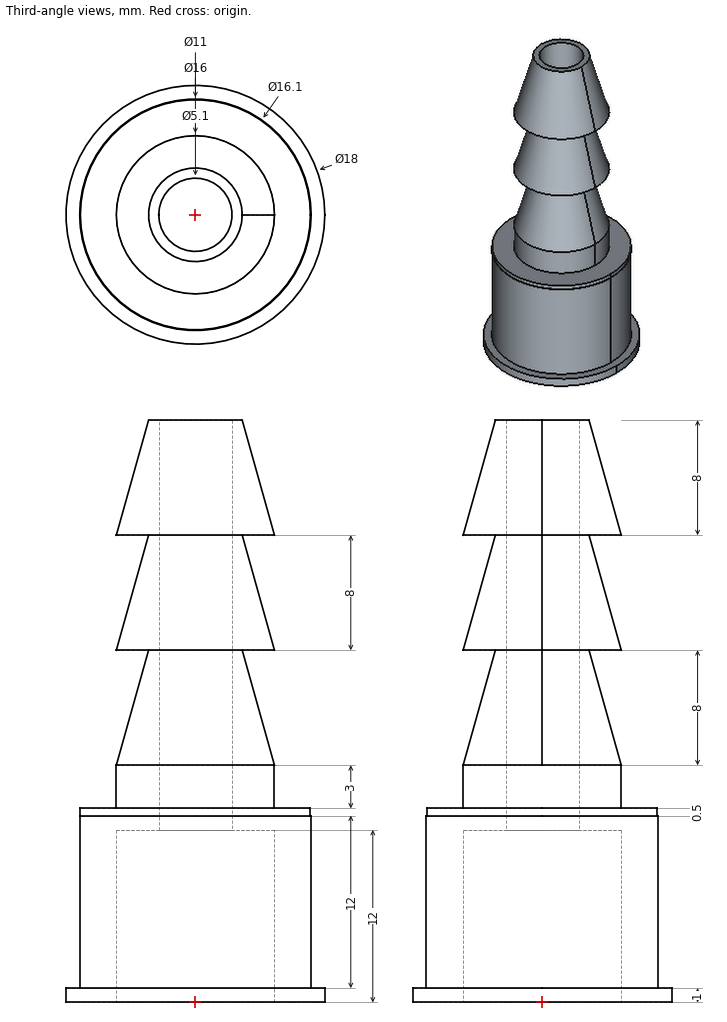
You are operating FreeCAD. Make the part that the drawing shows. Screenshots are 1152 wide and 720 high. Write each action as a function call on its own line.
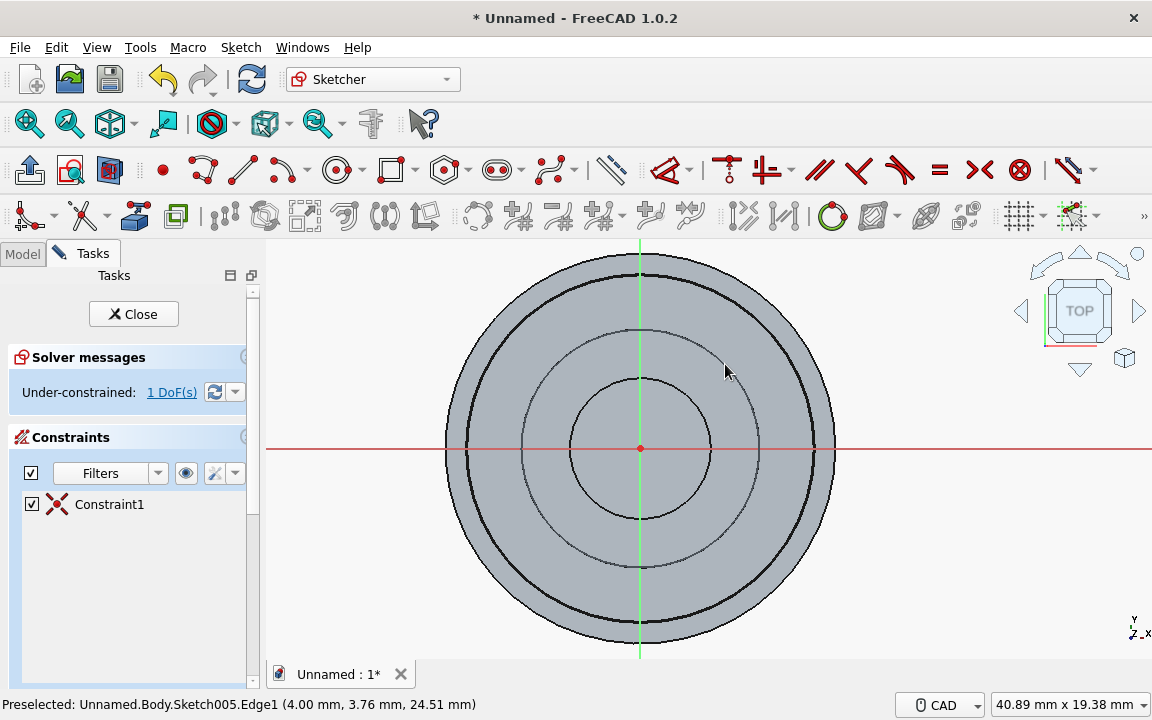
click(666, 170)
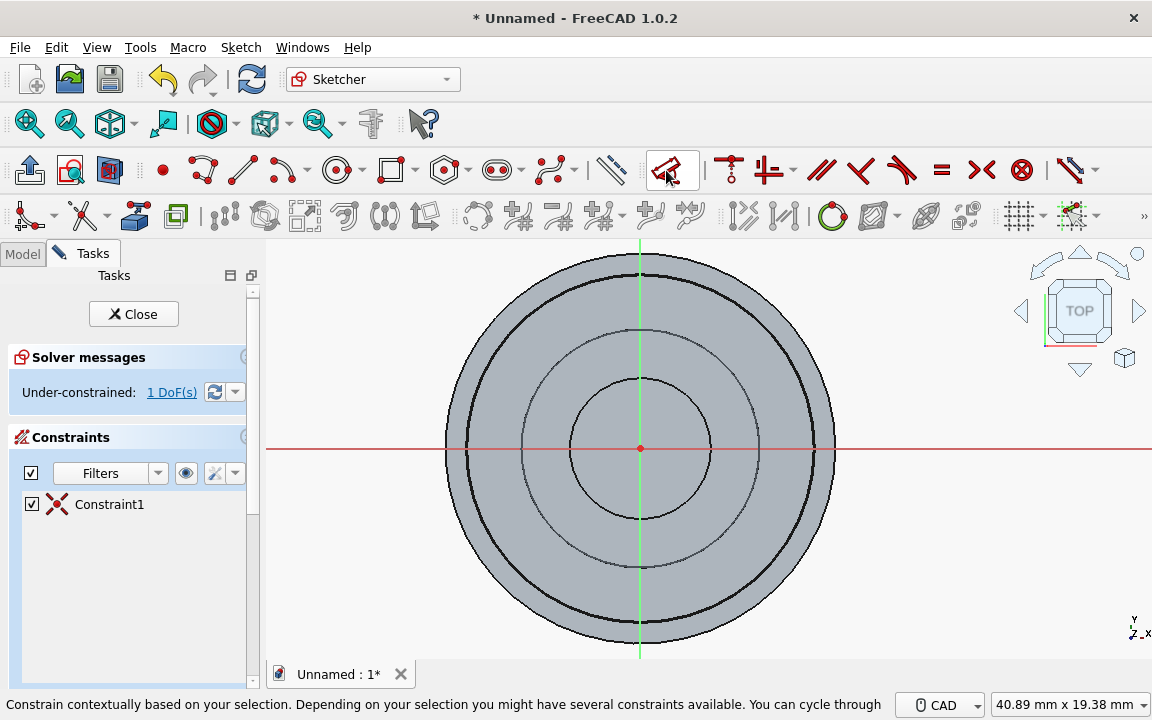
click(724, 364)
click(746, 341)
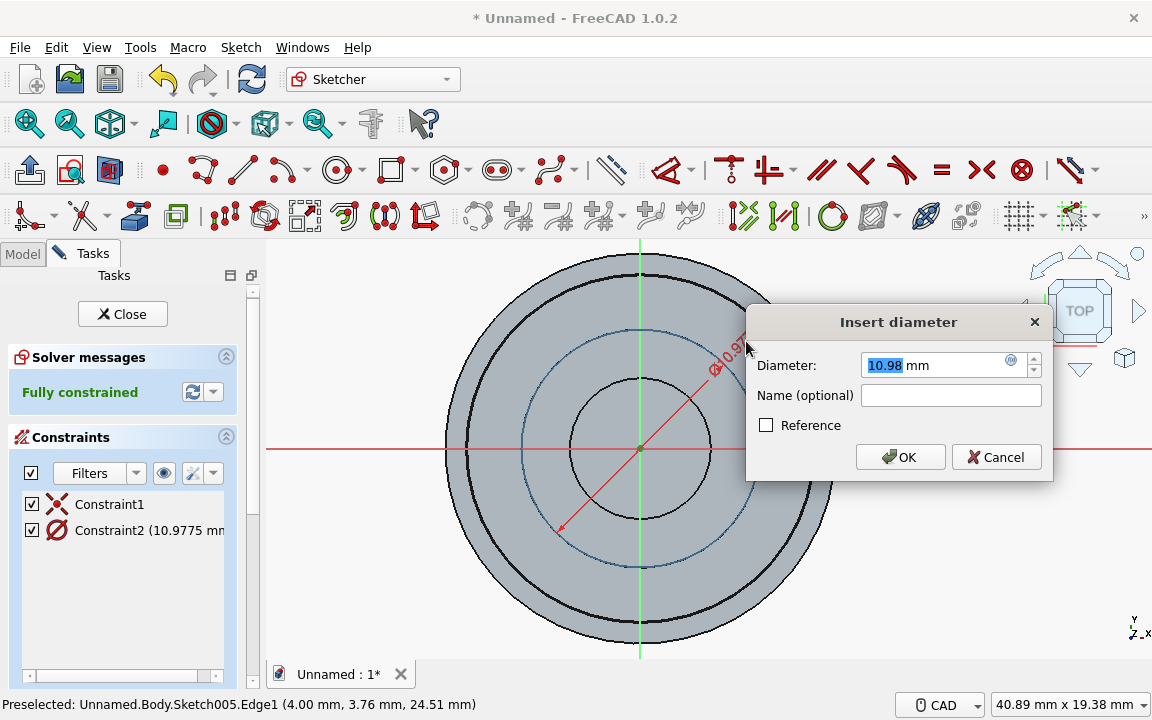
text(11)
key(Return)
key(Escape)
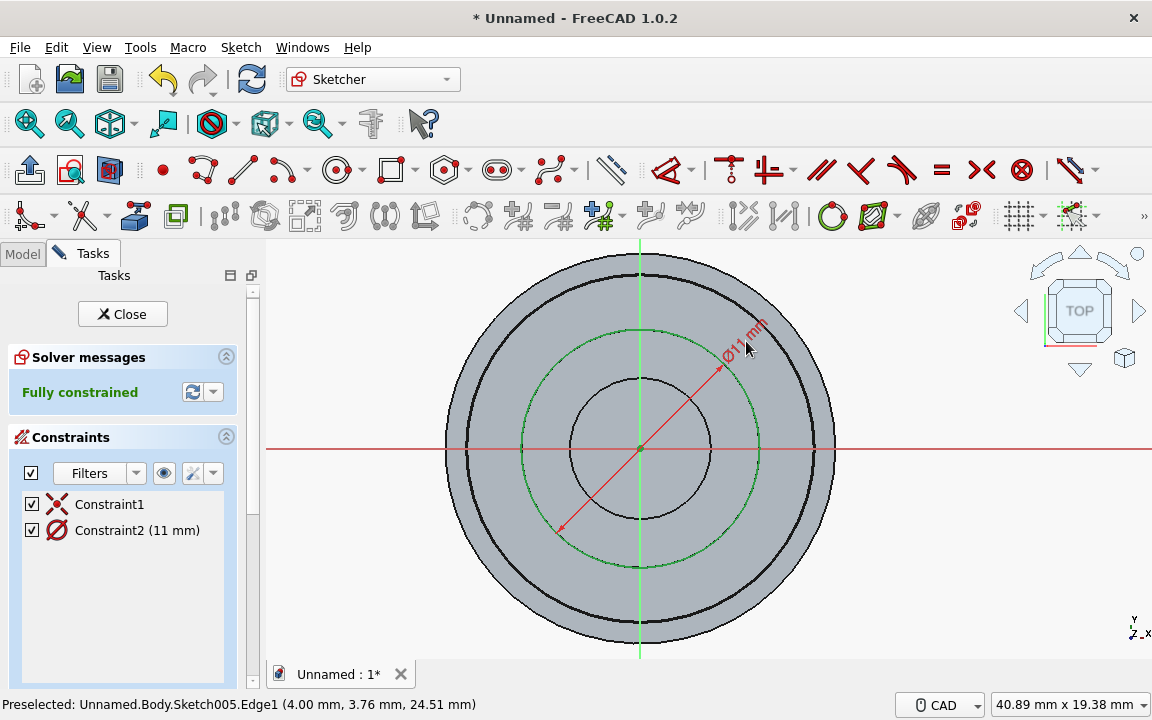
click(123, 314)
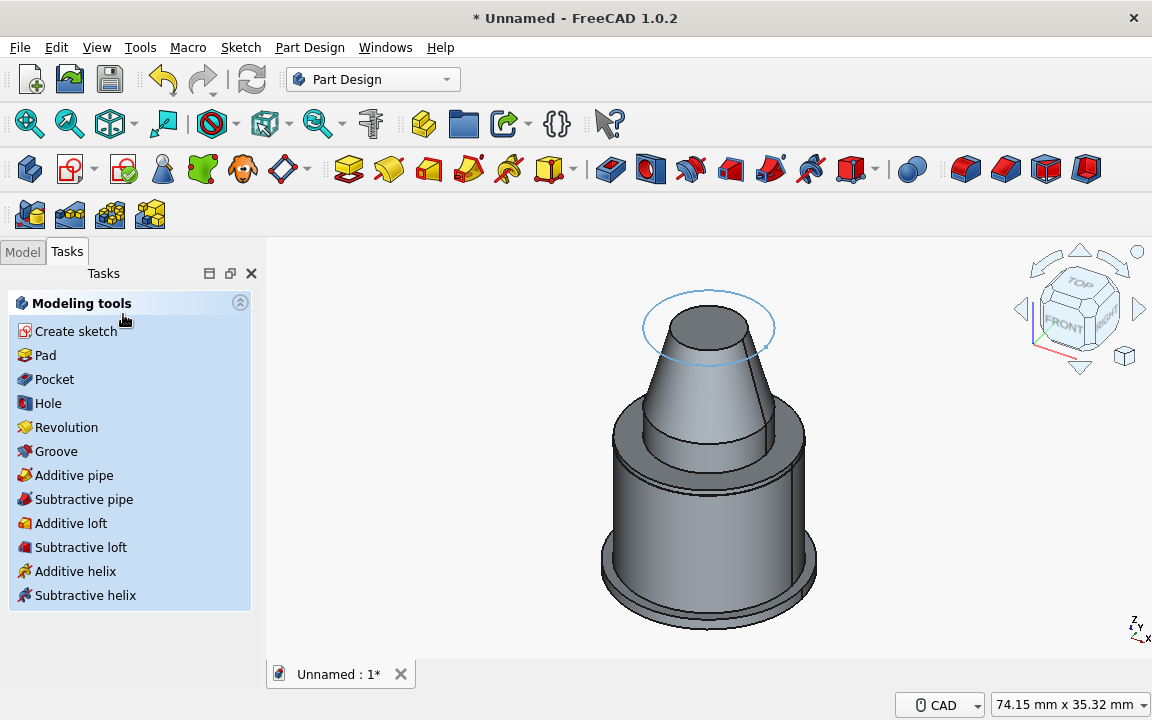
click(350, 170)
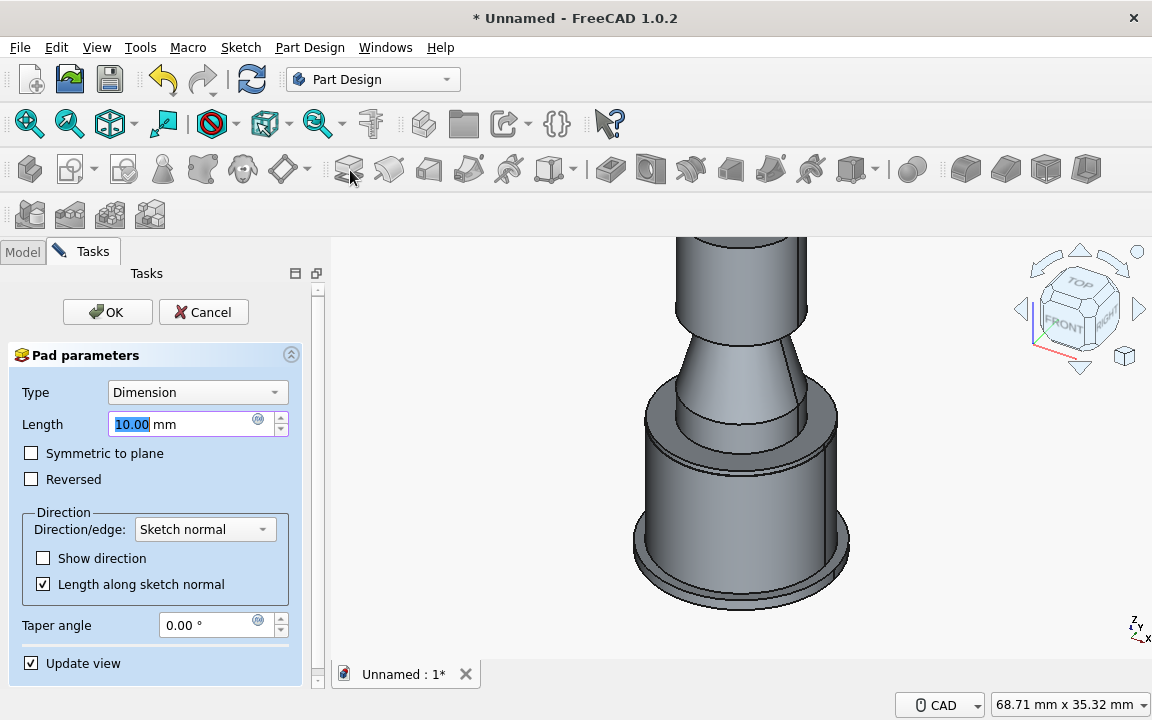
text(8)
key(Tab)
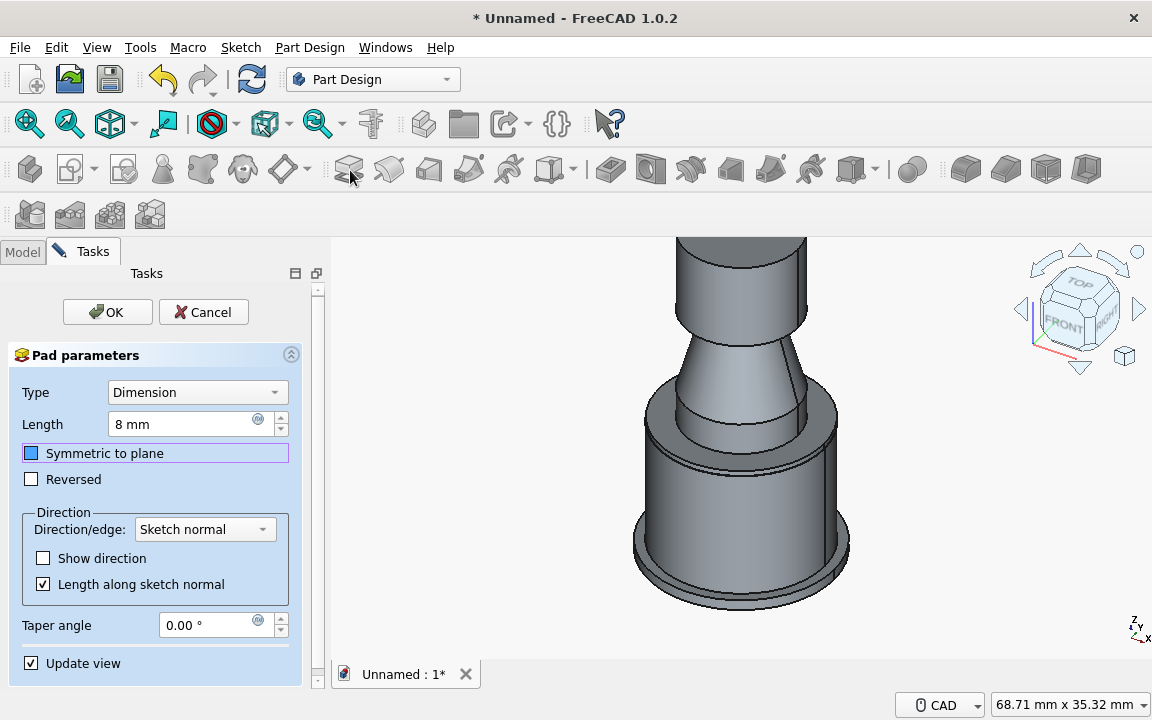
triple_click(216, 625)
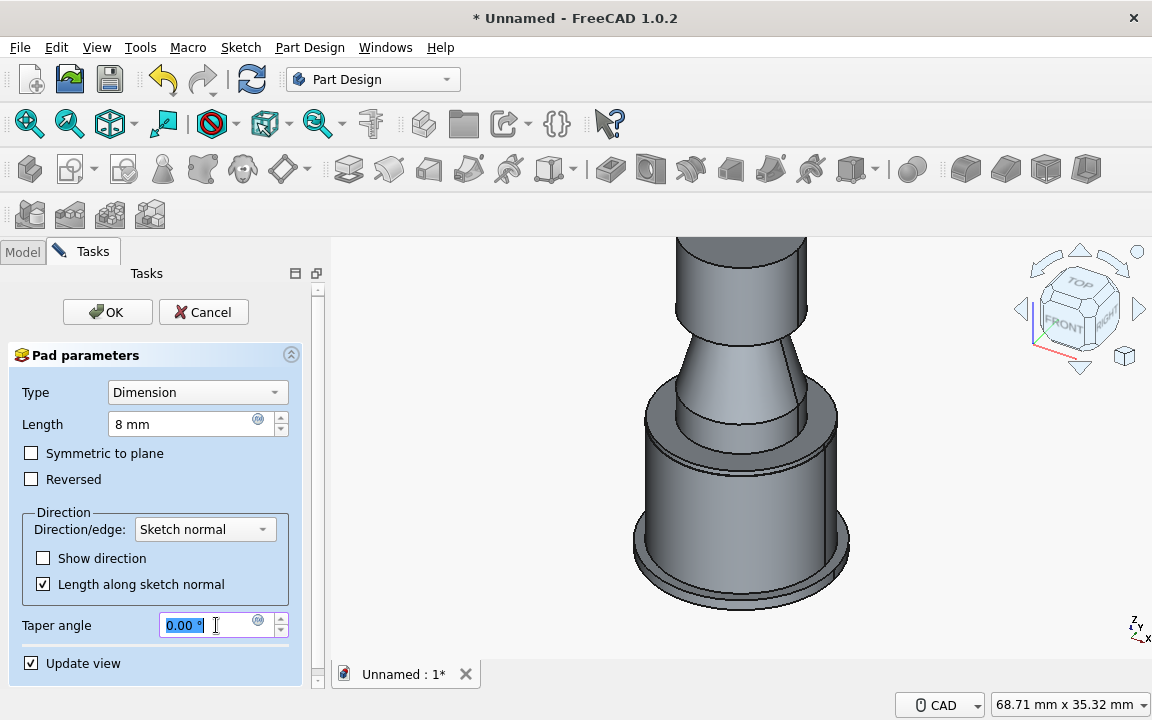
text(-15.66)
key(Tab)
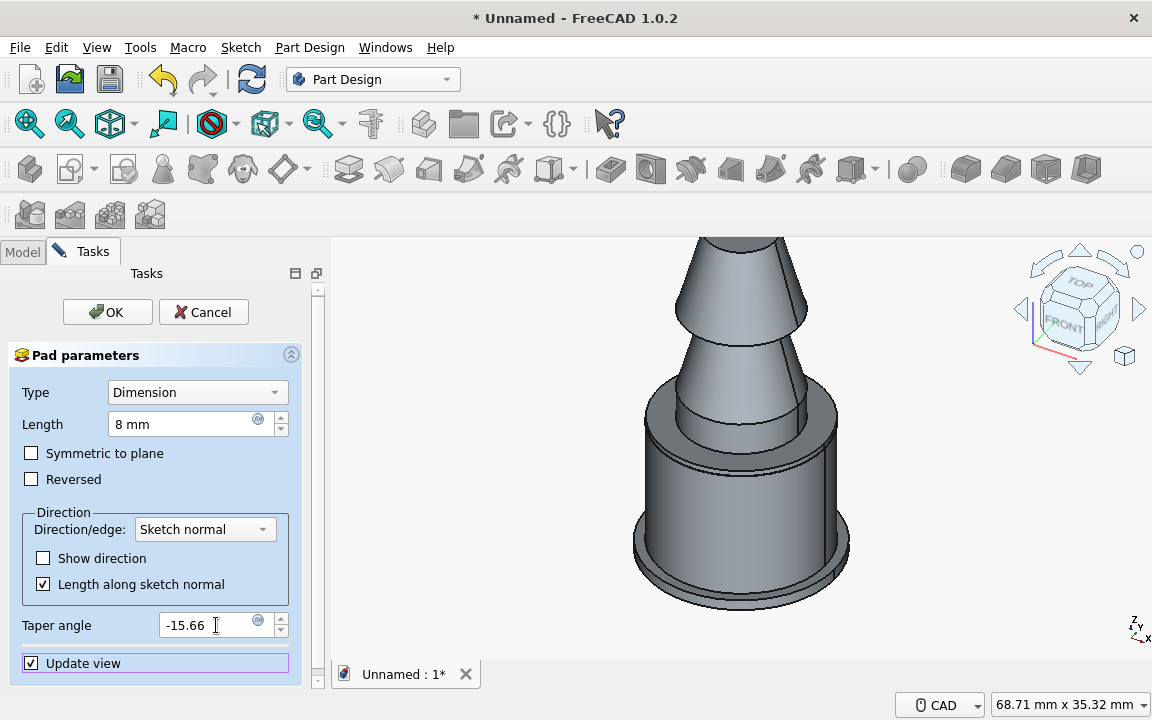
click(108, 312)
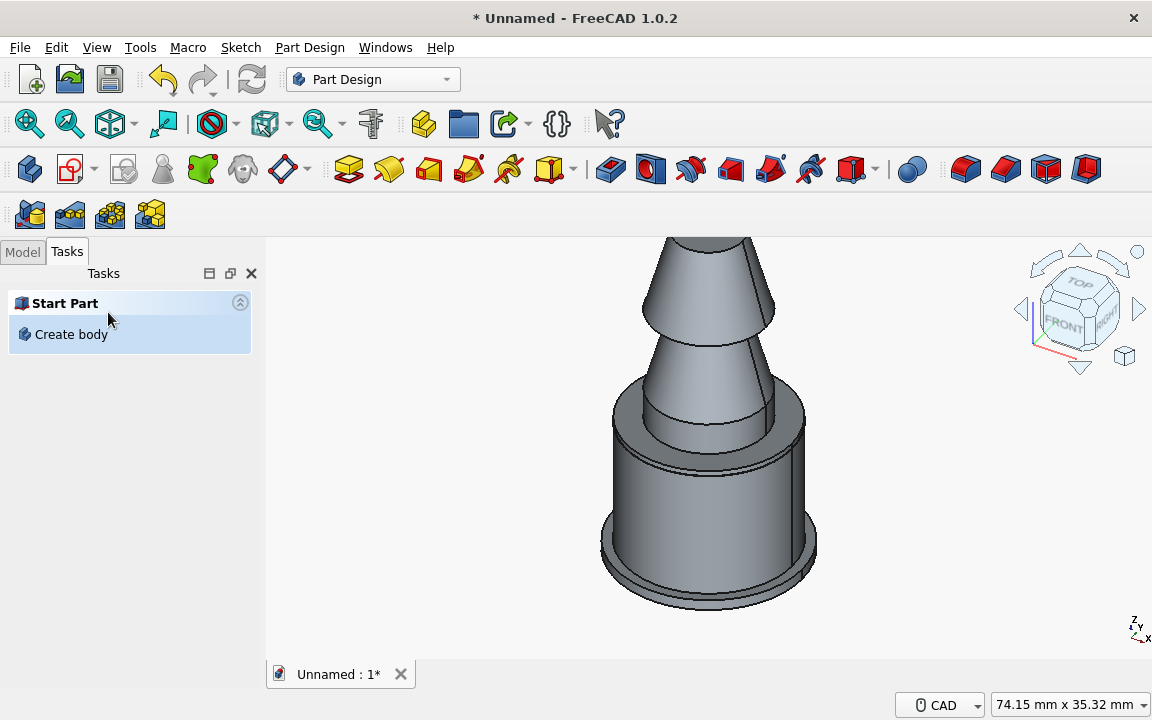
key(v)
key(f)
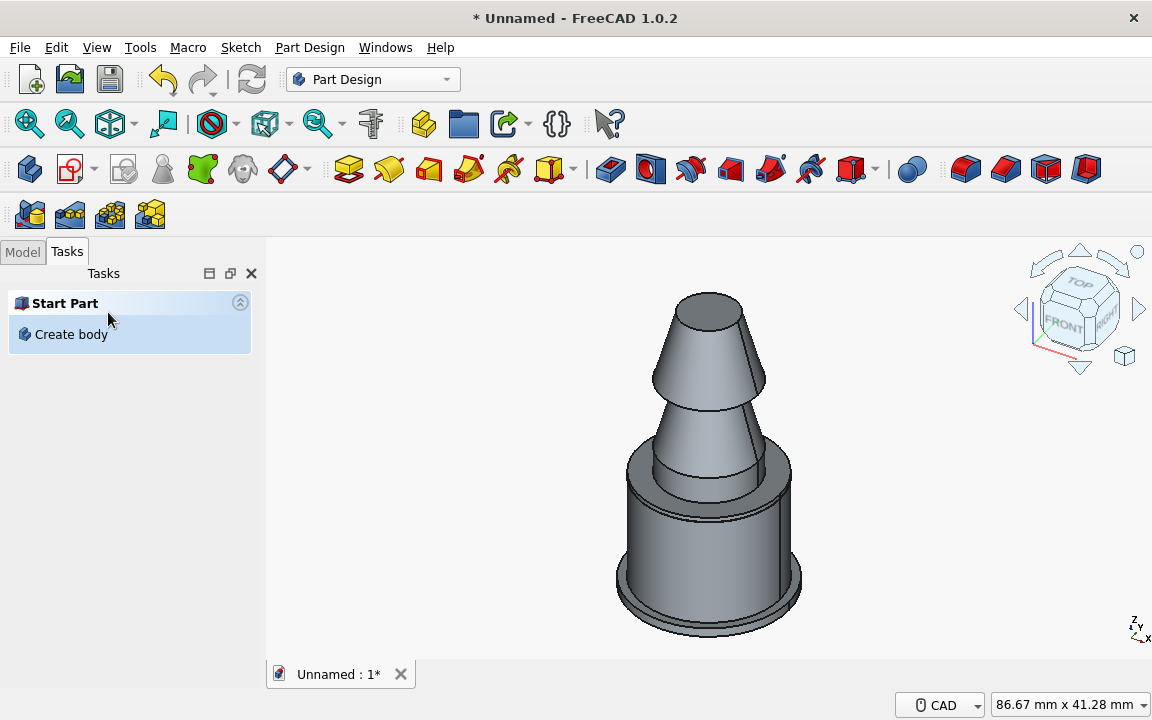
click(709, 311)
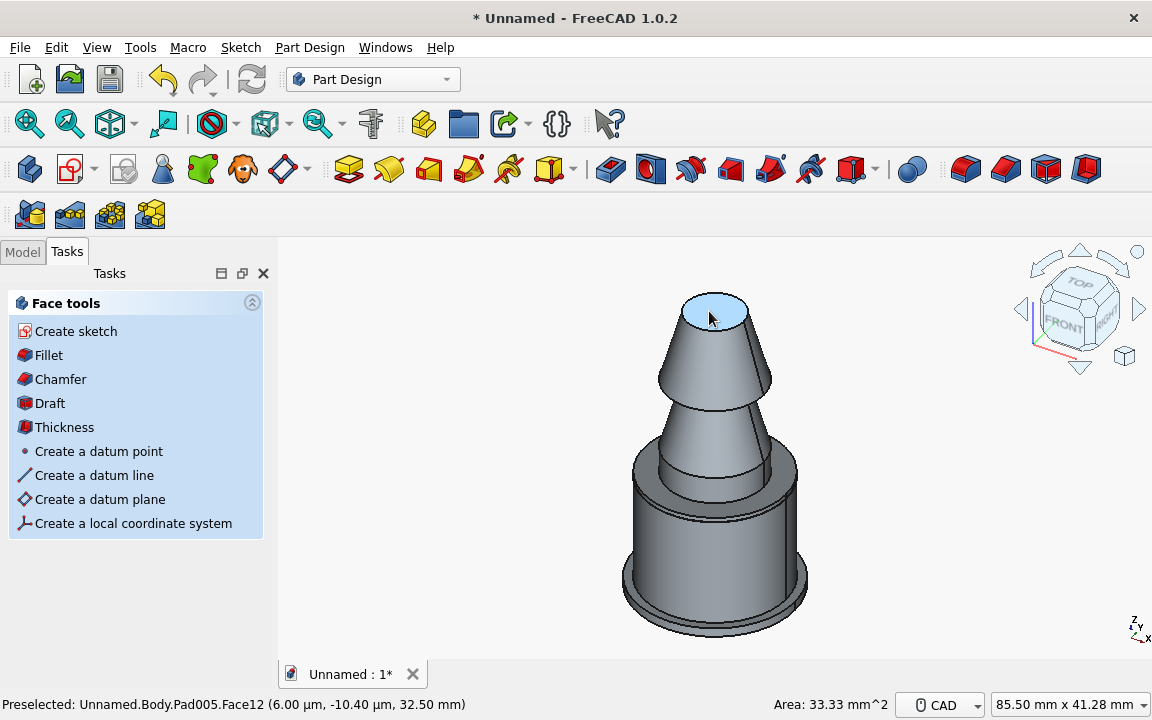
click(70, 170)